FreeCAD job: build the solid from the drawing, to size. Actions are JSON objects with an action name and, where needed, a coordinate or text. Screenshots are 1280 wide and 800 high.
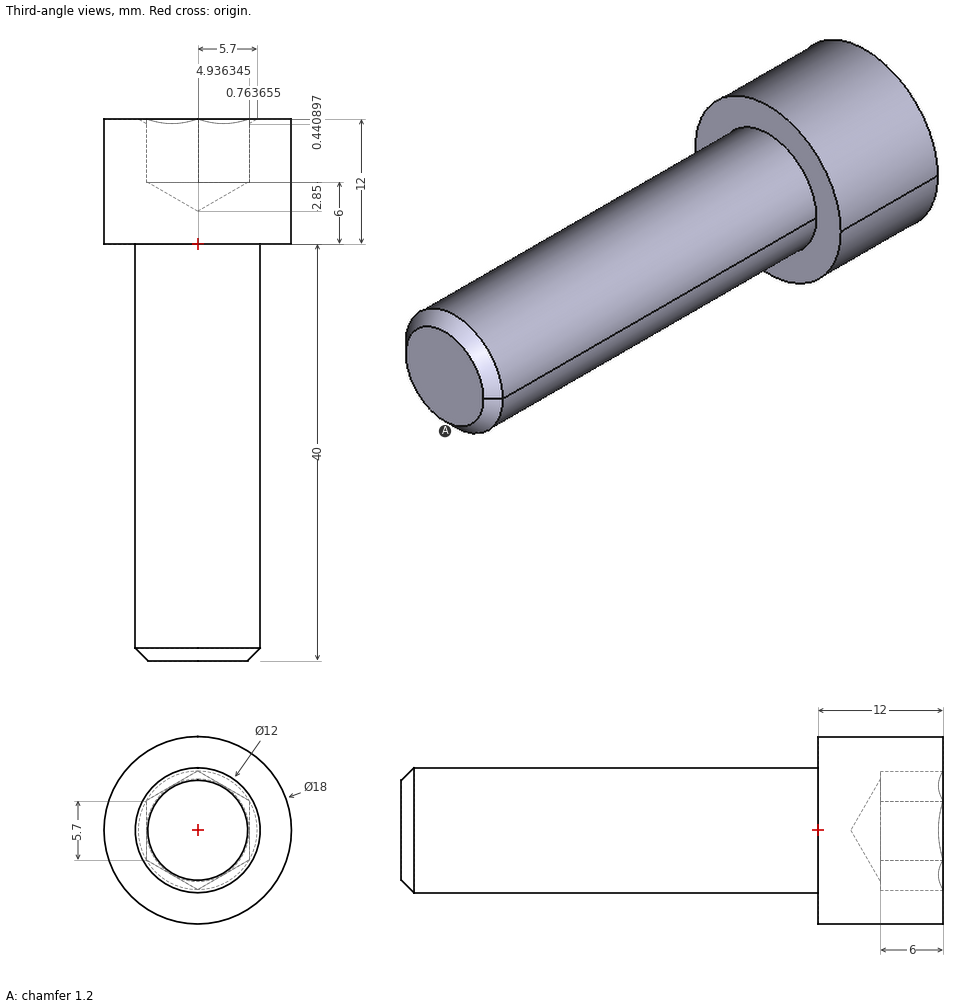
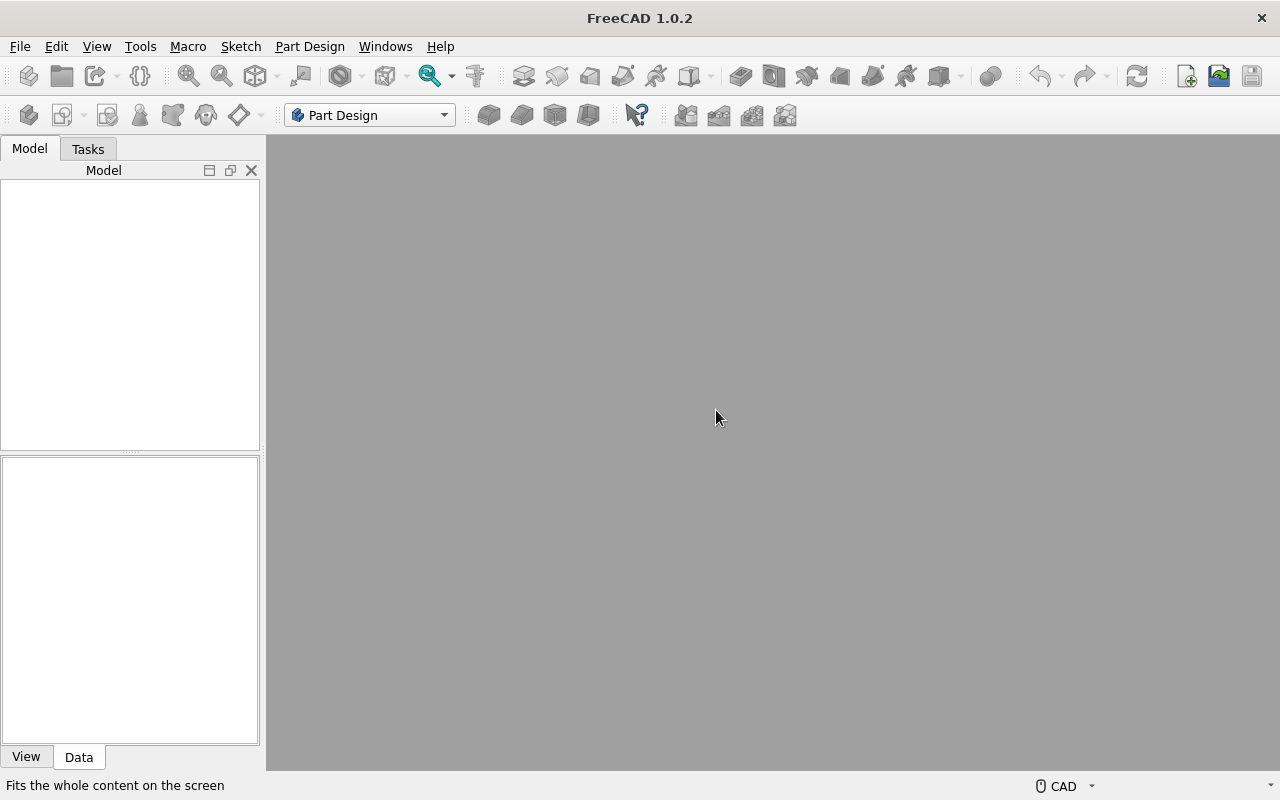
{"action": "left_click", "coordinate": [1186, 76]}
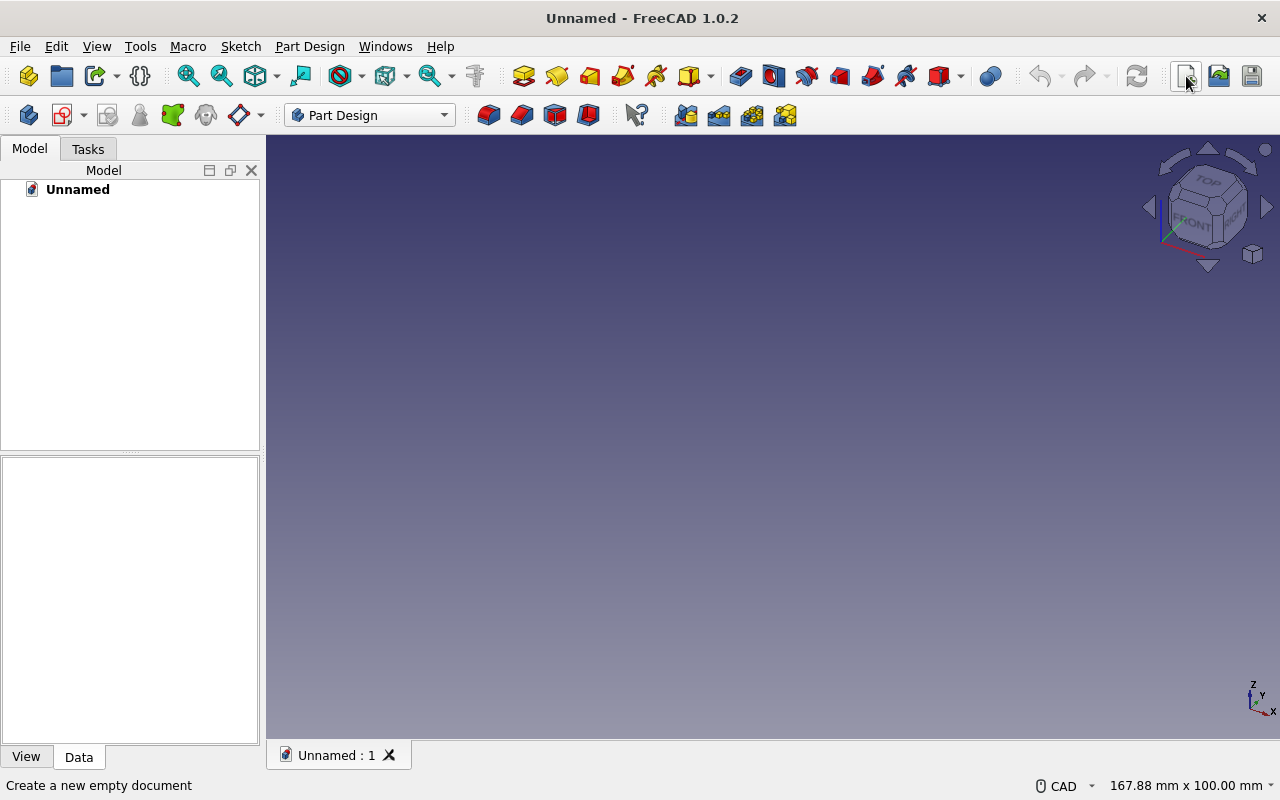
{"action": "left_click", "coordinate": [62, 116]}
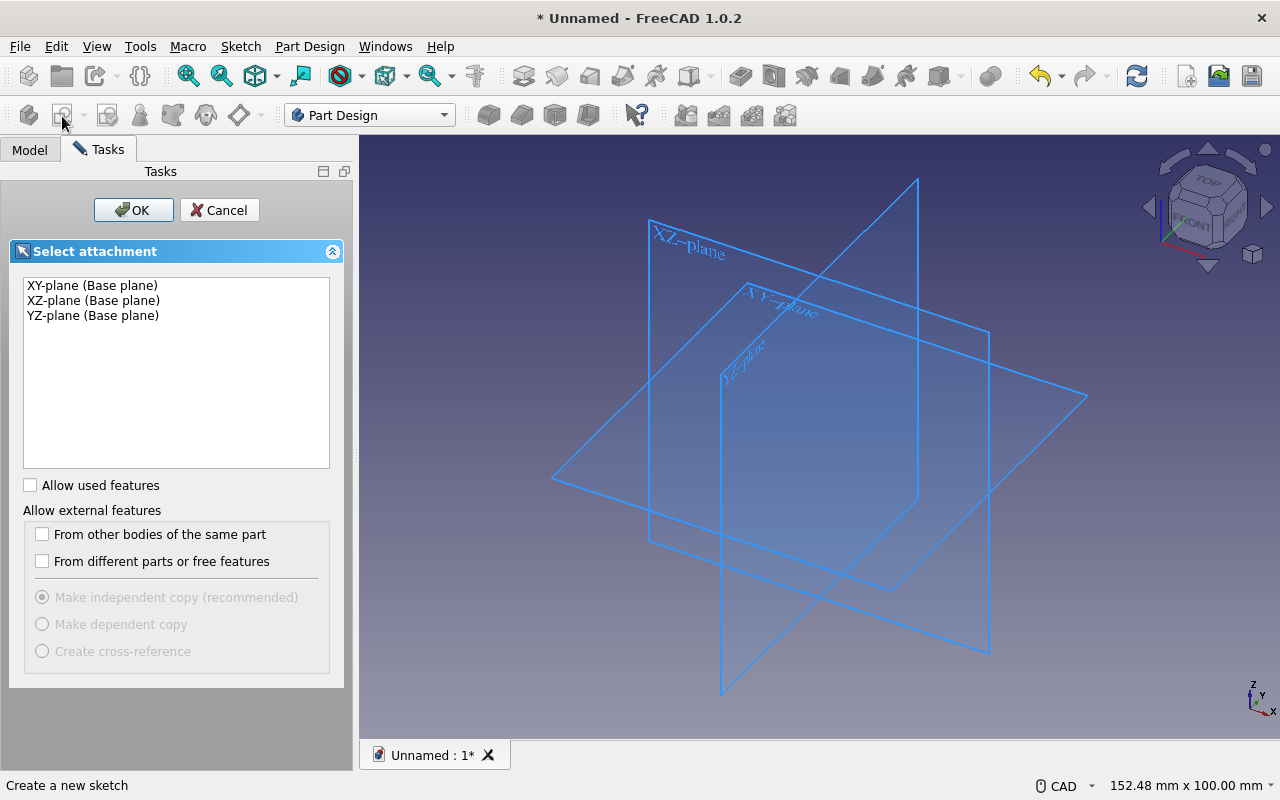
{"action": "left_click", "coordinate": [84, 300]}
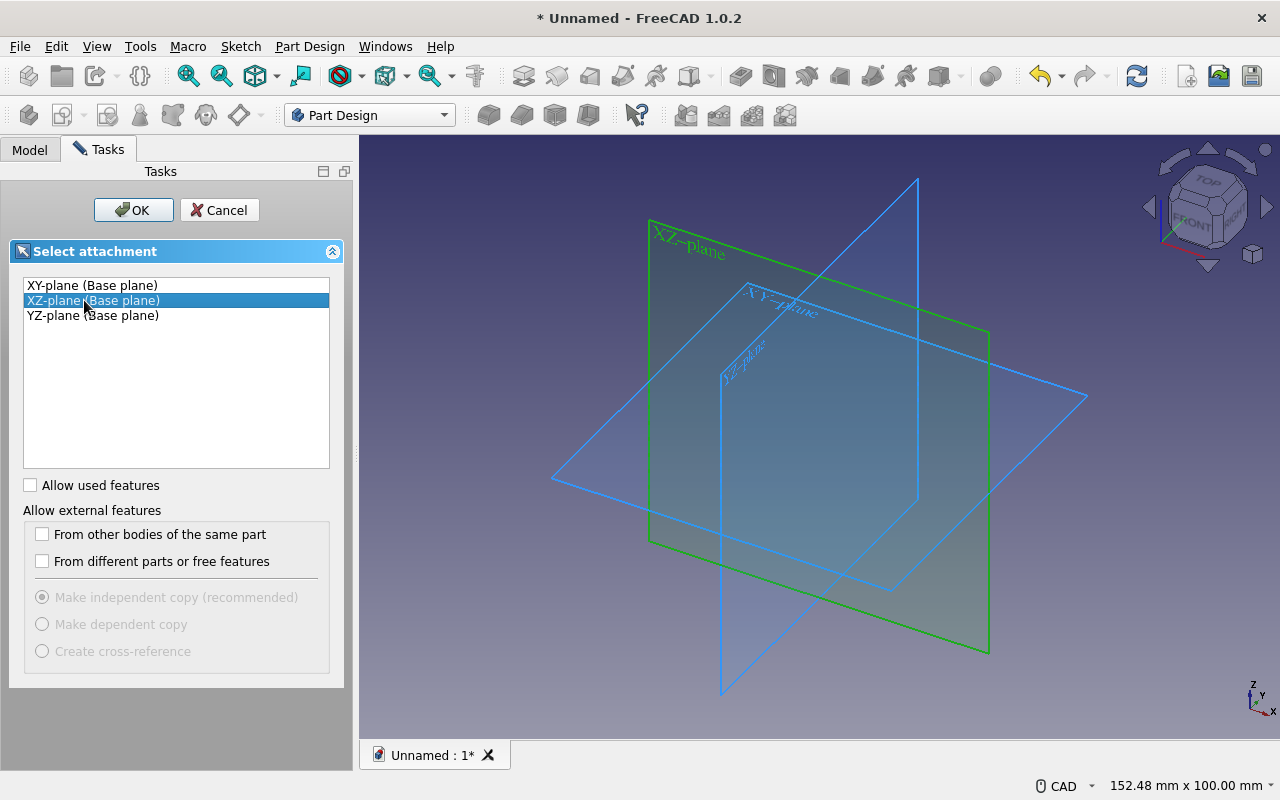
{"action": "left_click", "coordinate": [134, 210]}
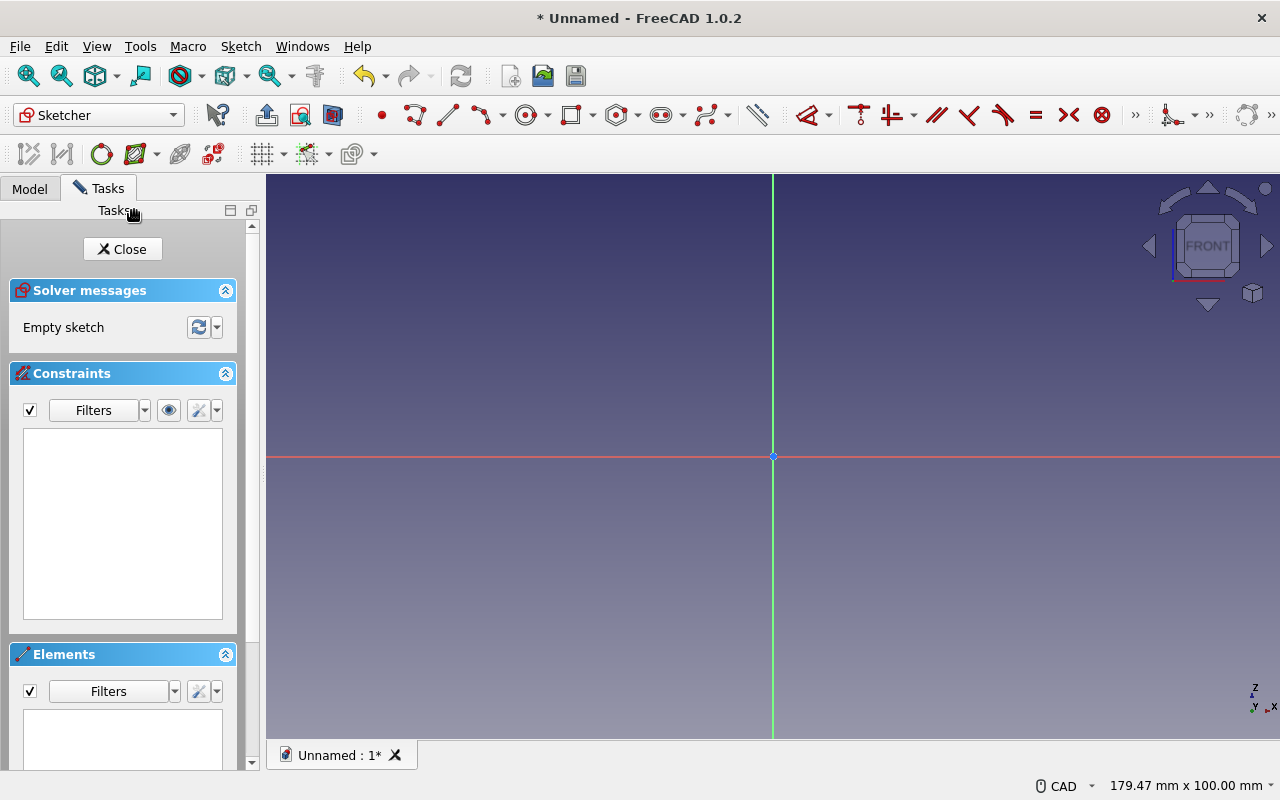
{"action": "scroll", "coordinate": [803, 456], "scroll_direction": "up", "scroll_amount": 6}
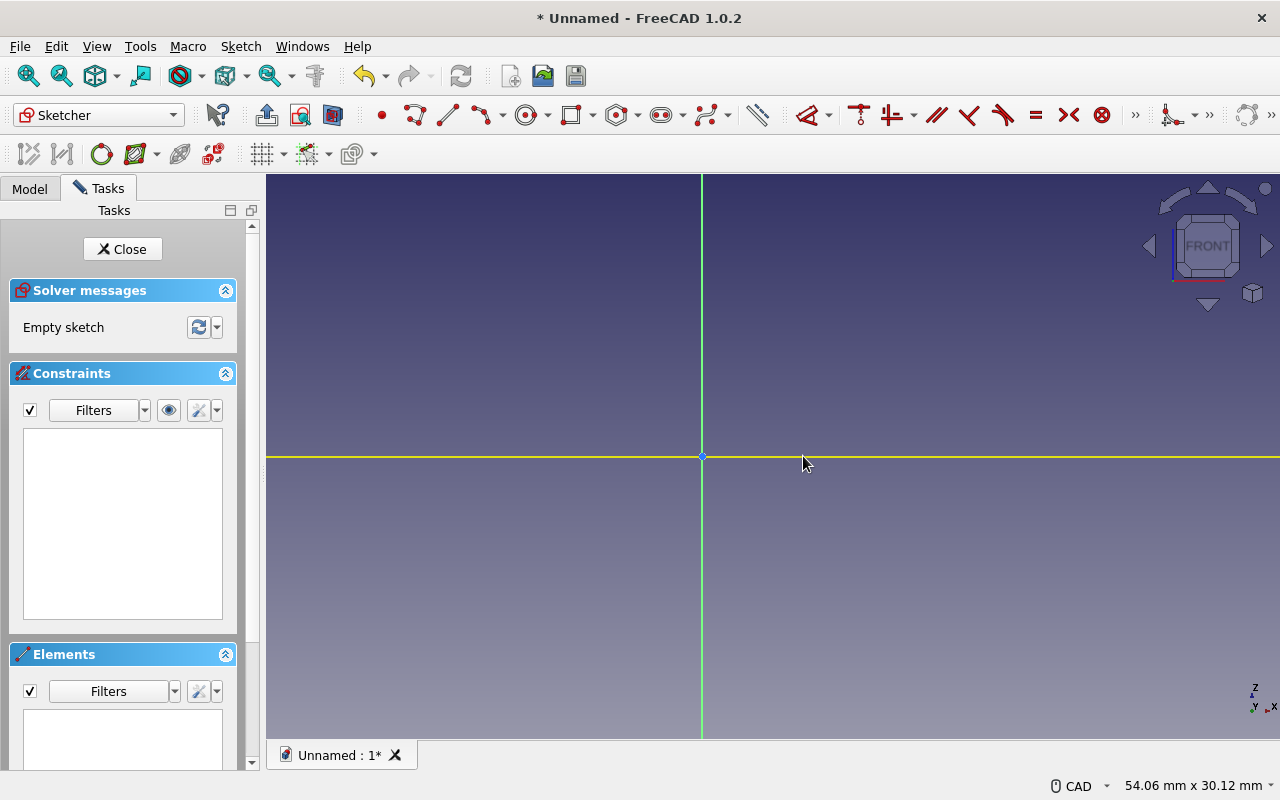
{"action": "left_click", "coordinate": [526, 116]}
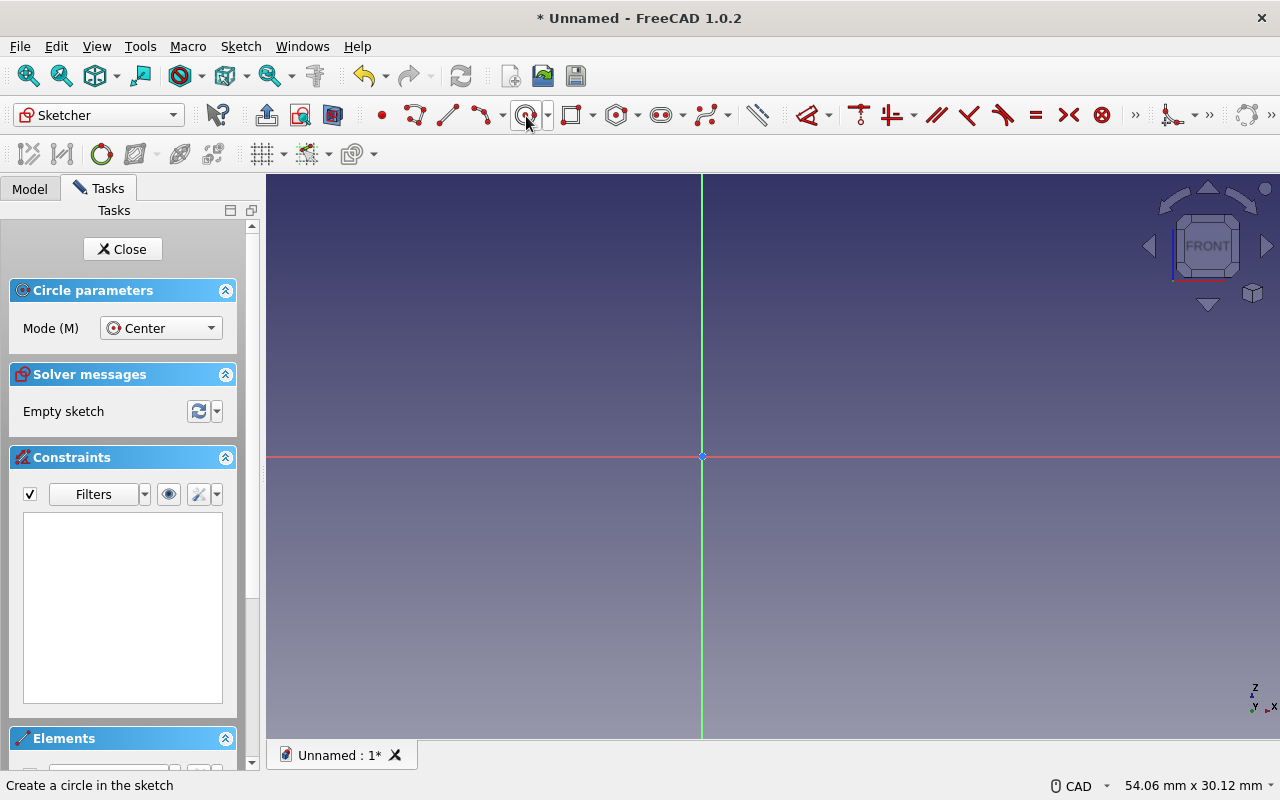
{"action": "left_click", "coordinate": [702, 456]}
{"action": "mouse_move", "coordinate": [822, 337]}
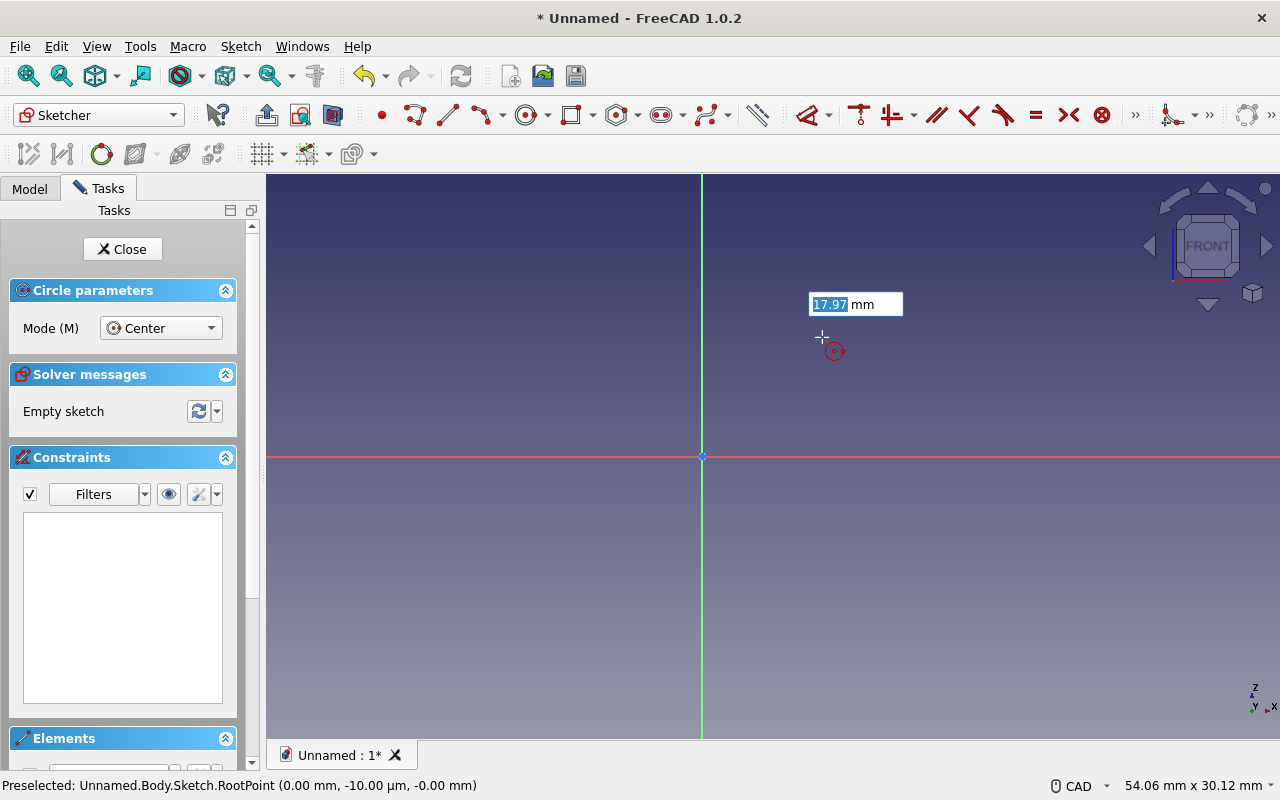
{"action": "type", "text": "18"}
{"action": "key", "text": "Return"}
{"action": "key", "text": "Escape"}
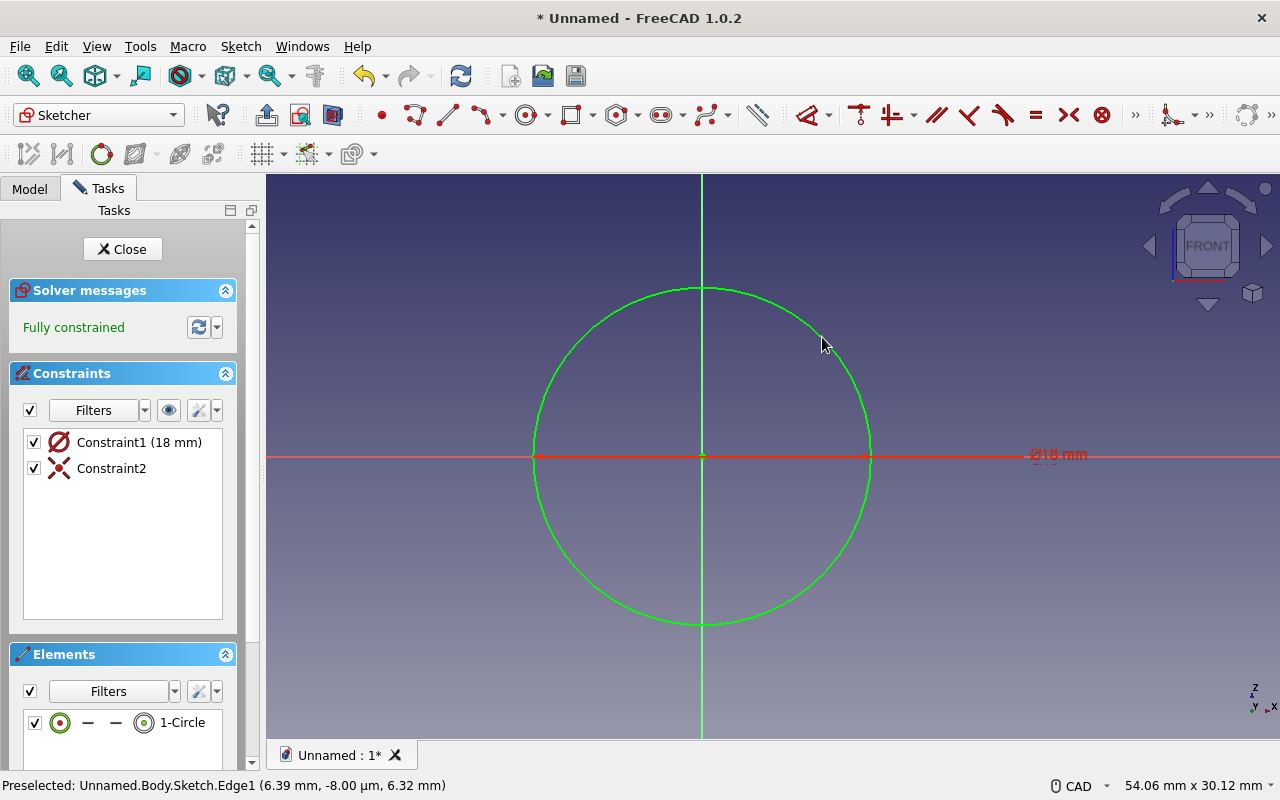
{"action": "left_click", "coordinate": [123, 249]}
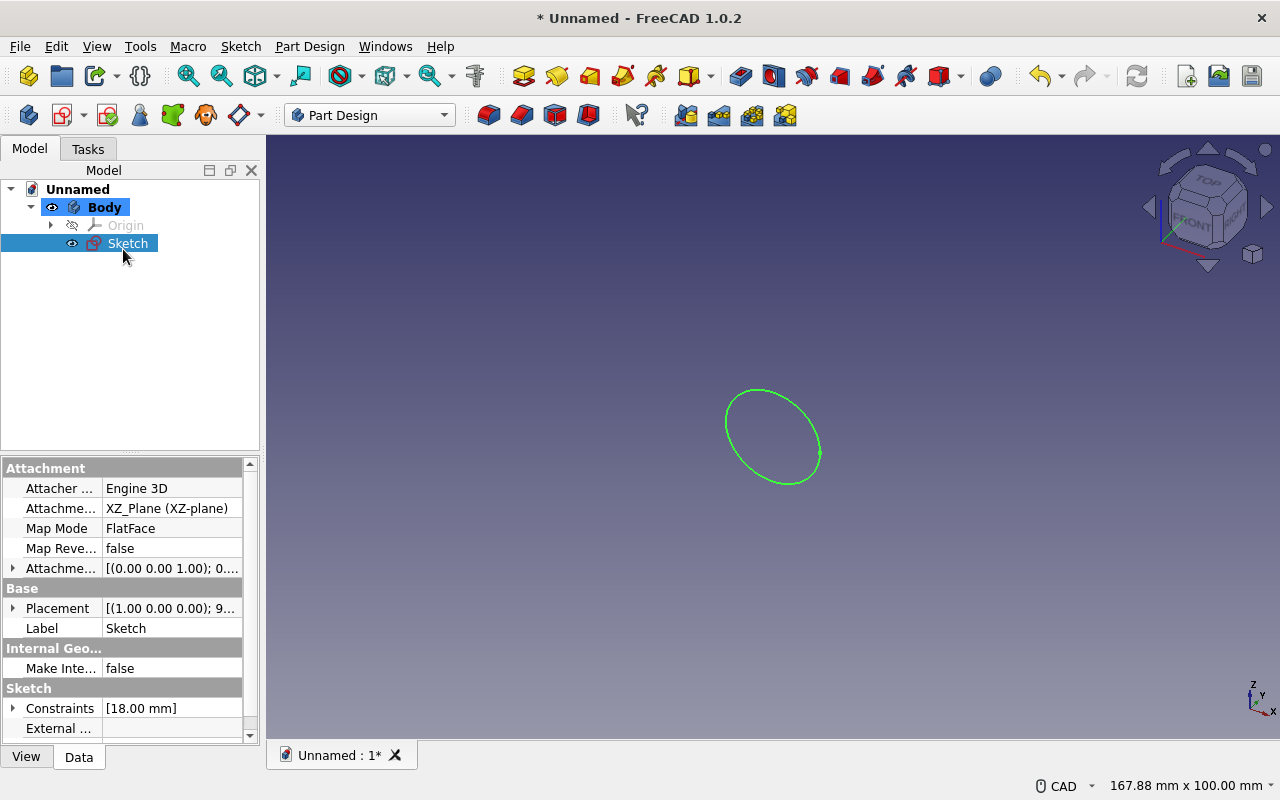
{"action": "left_click", "coordinate": [524, 76]}